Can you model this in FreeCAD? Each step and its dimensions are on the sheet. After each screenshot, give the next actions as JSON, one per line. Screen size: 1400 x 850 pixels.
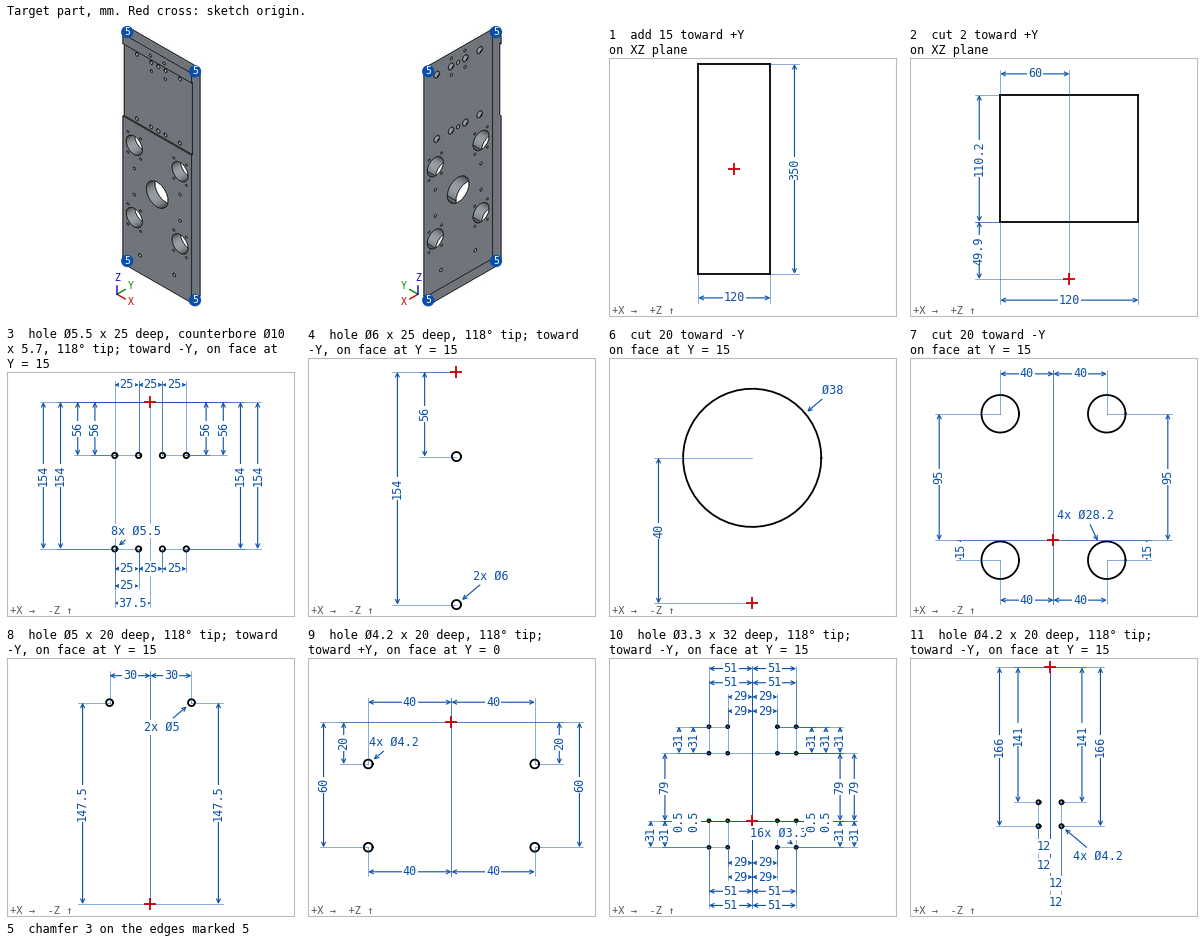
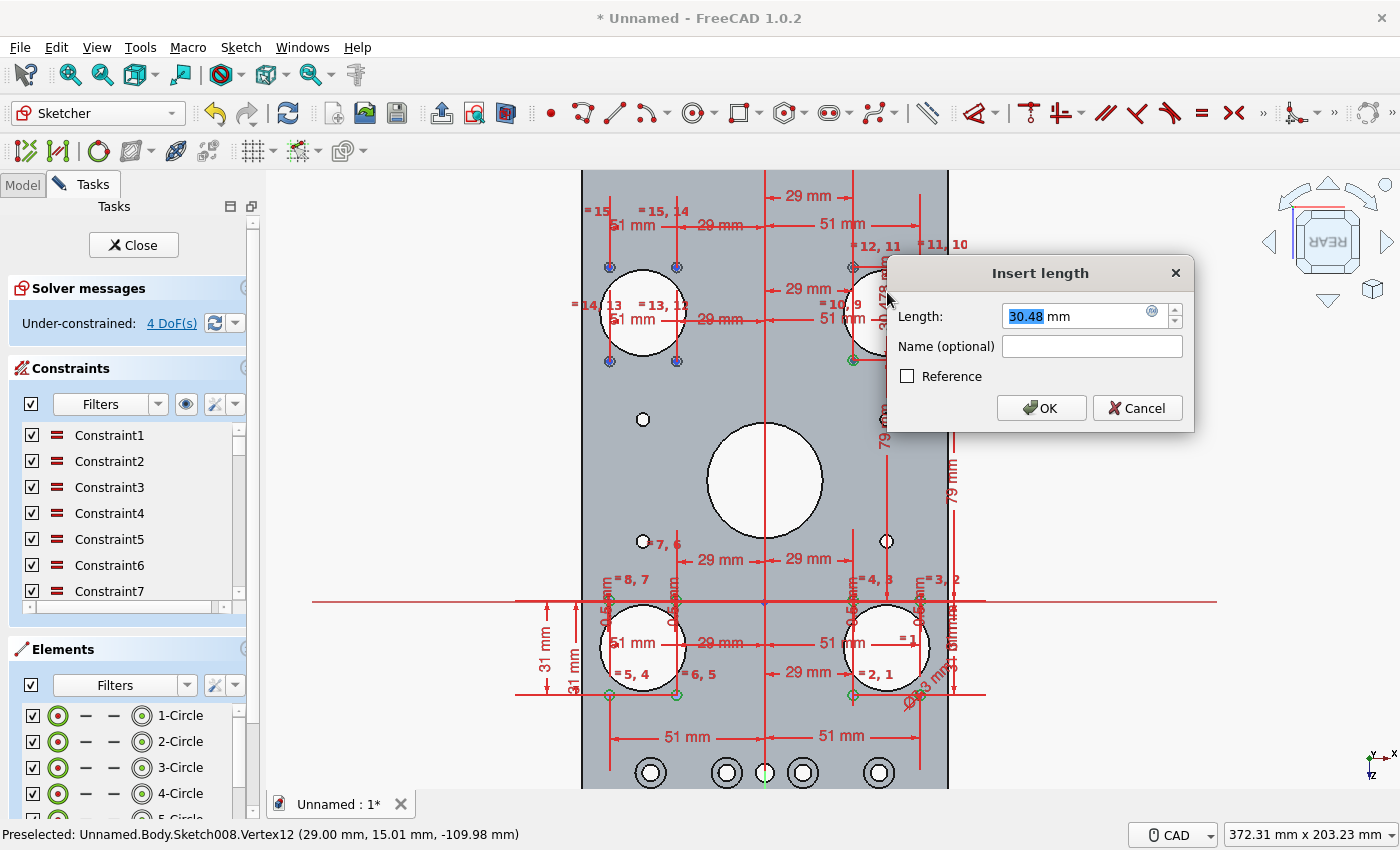
{"action": "type", "text": "31"}
{"action": "key", "text": "Return"}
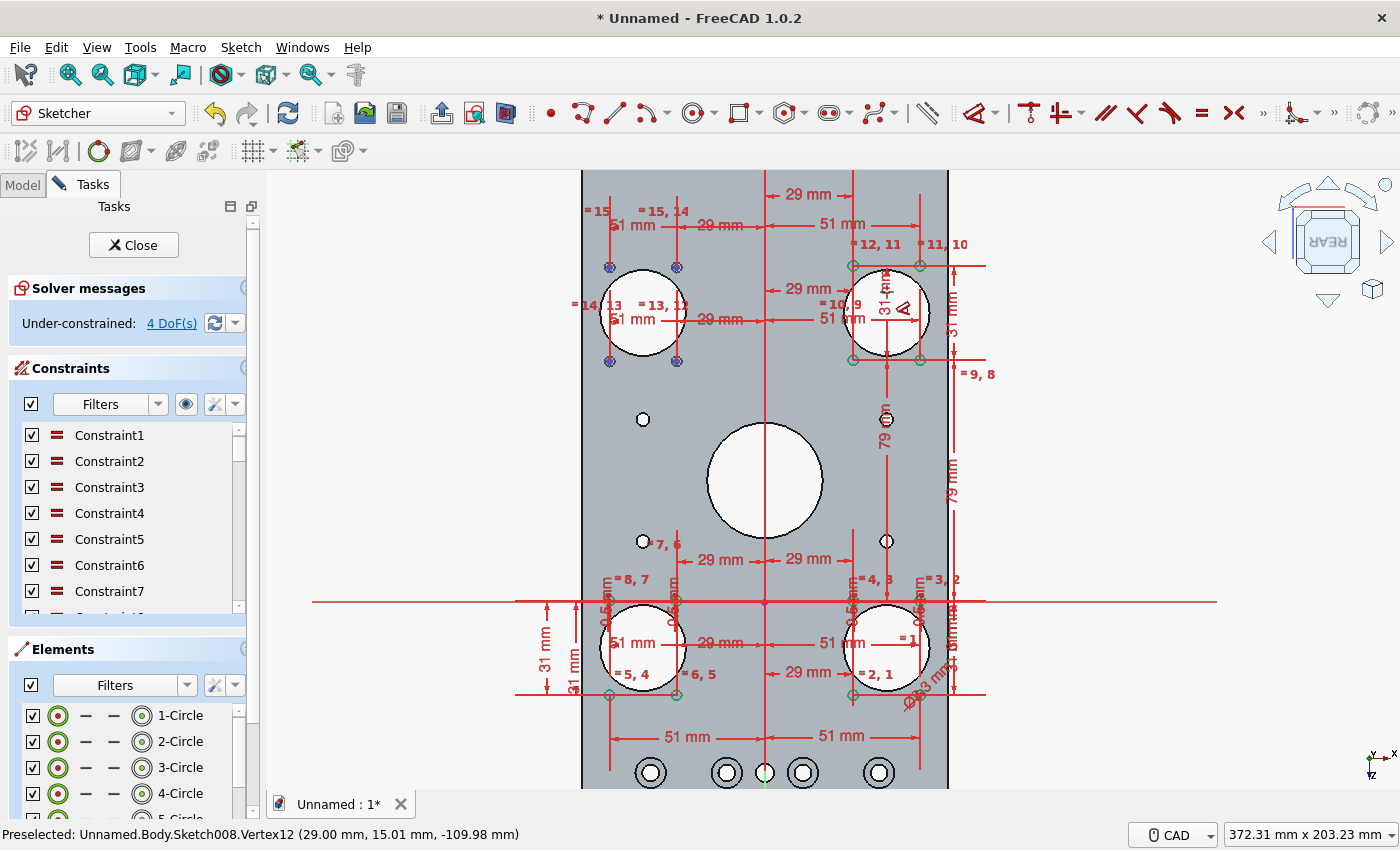
{"action": "left_click", "coordinate": [853, 266]}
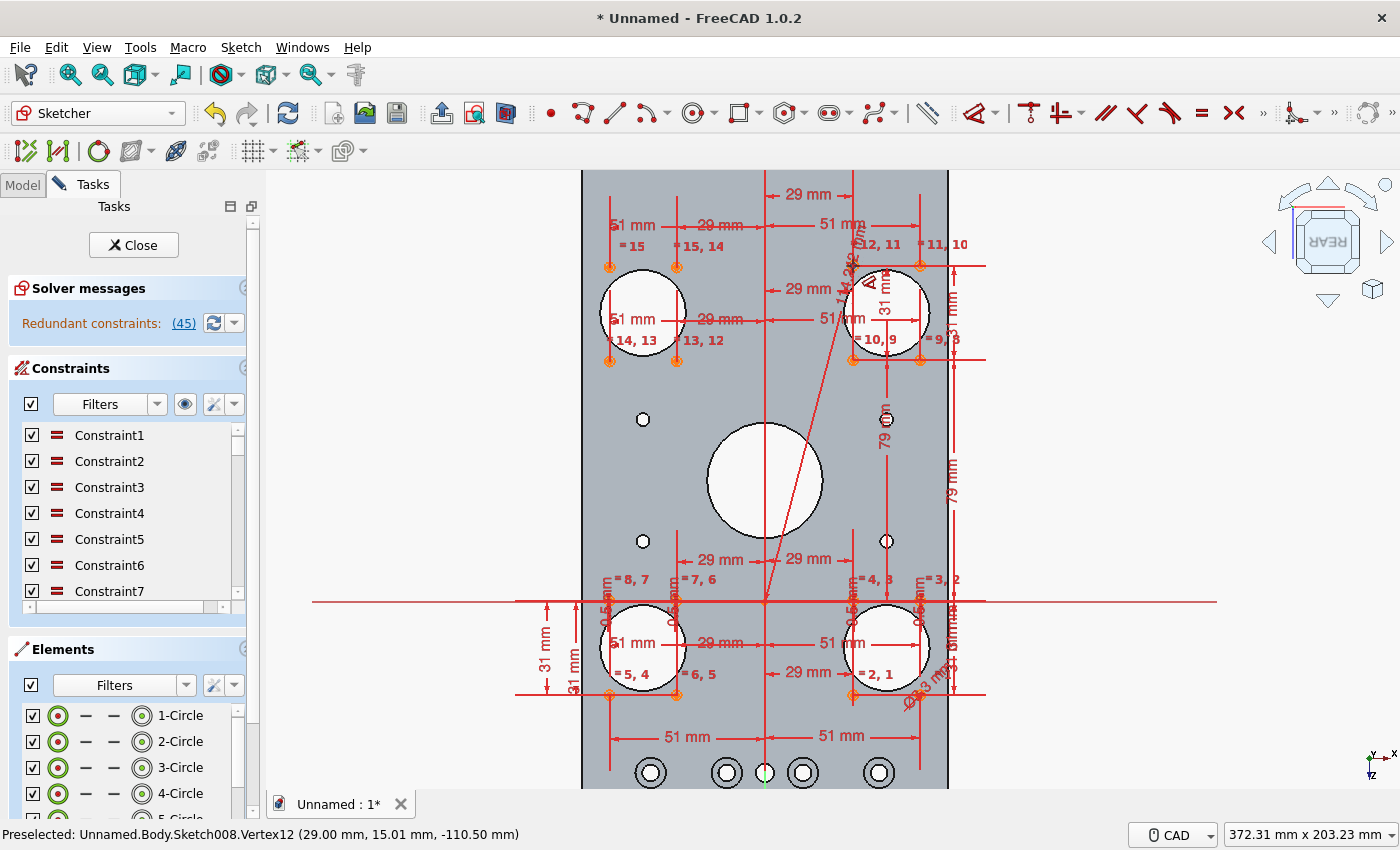
{"action": "left_click", "coordinate": [677, 361]}
{"action": "left_click", "coordinate": [887, 347]}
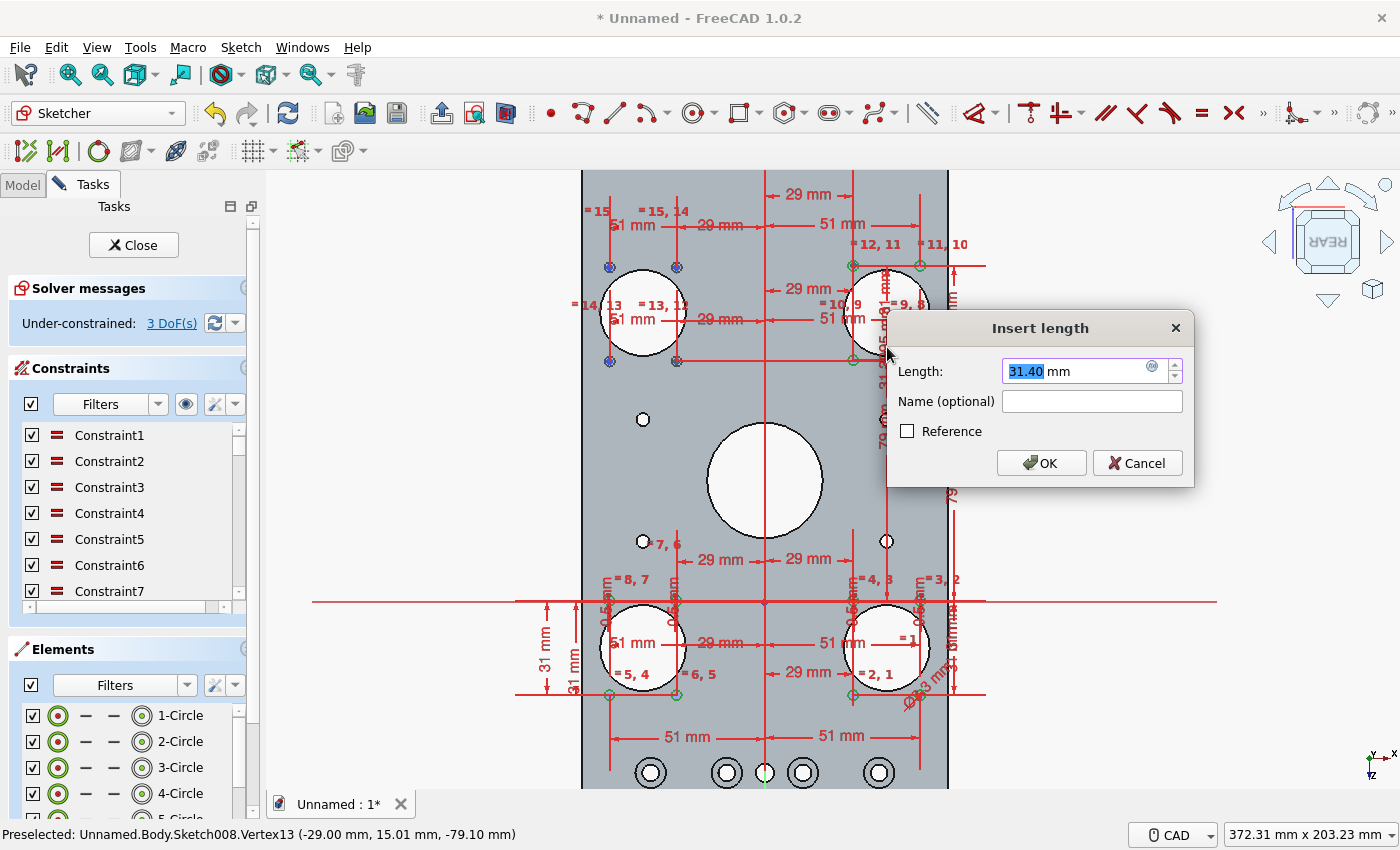
{"action": "type", "text": "31"}
{"action": "key", "text": "Return"}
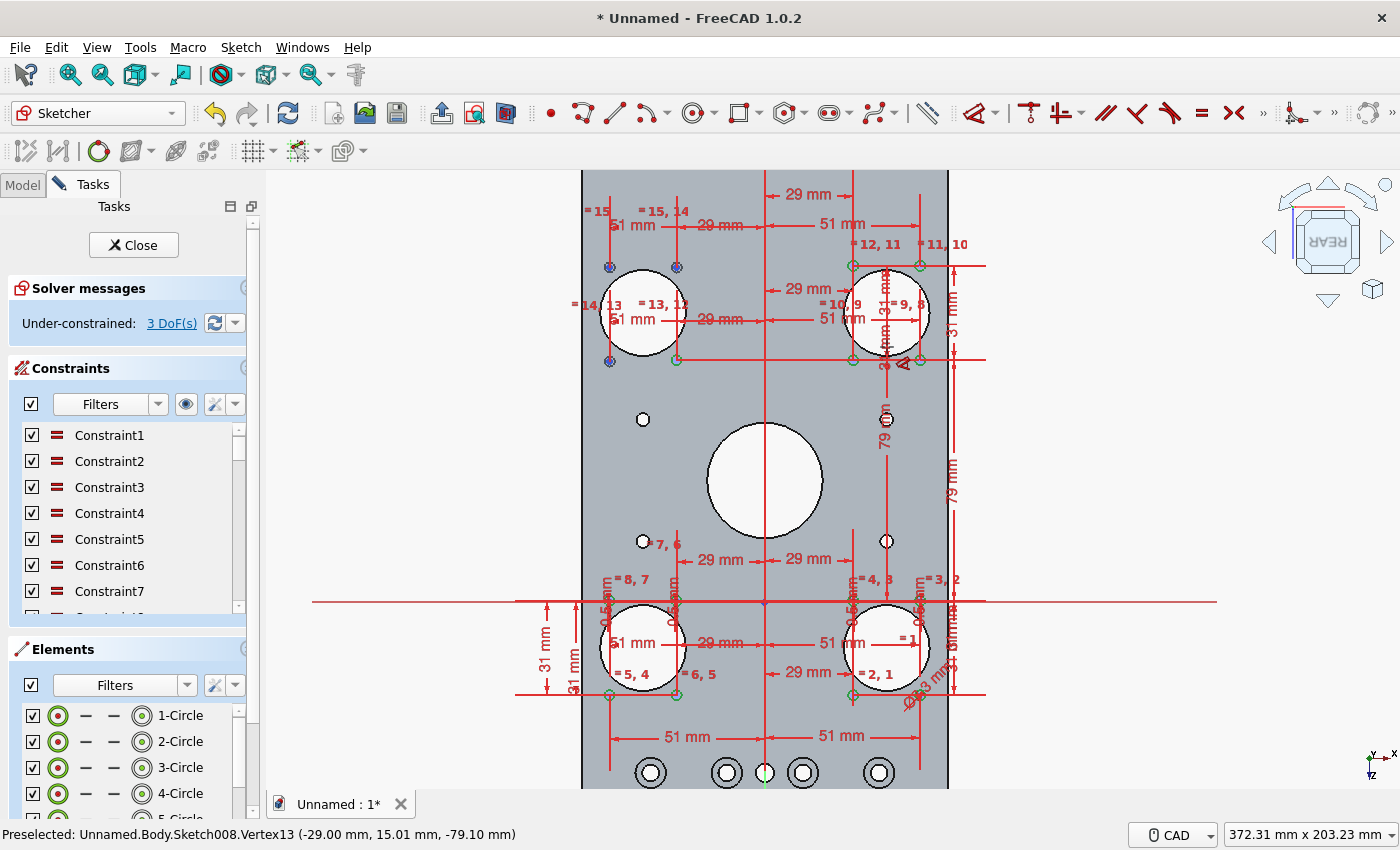
{"action": "left_click", "coordinate": [610, 601]}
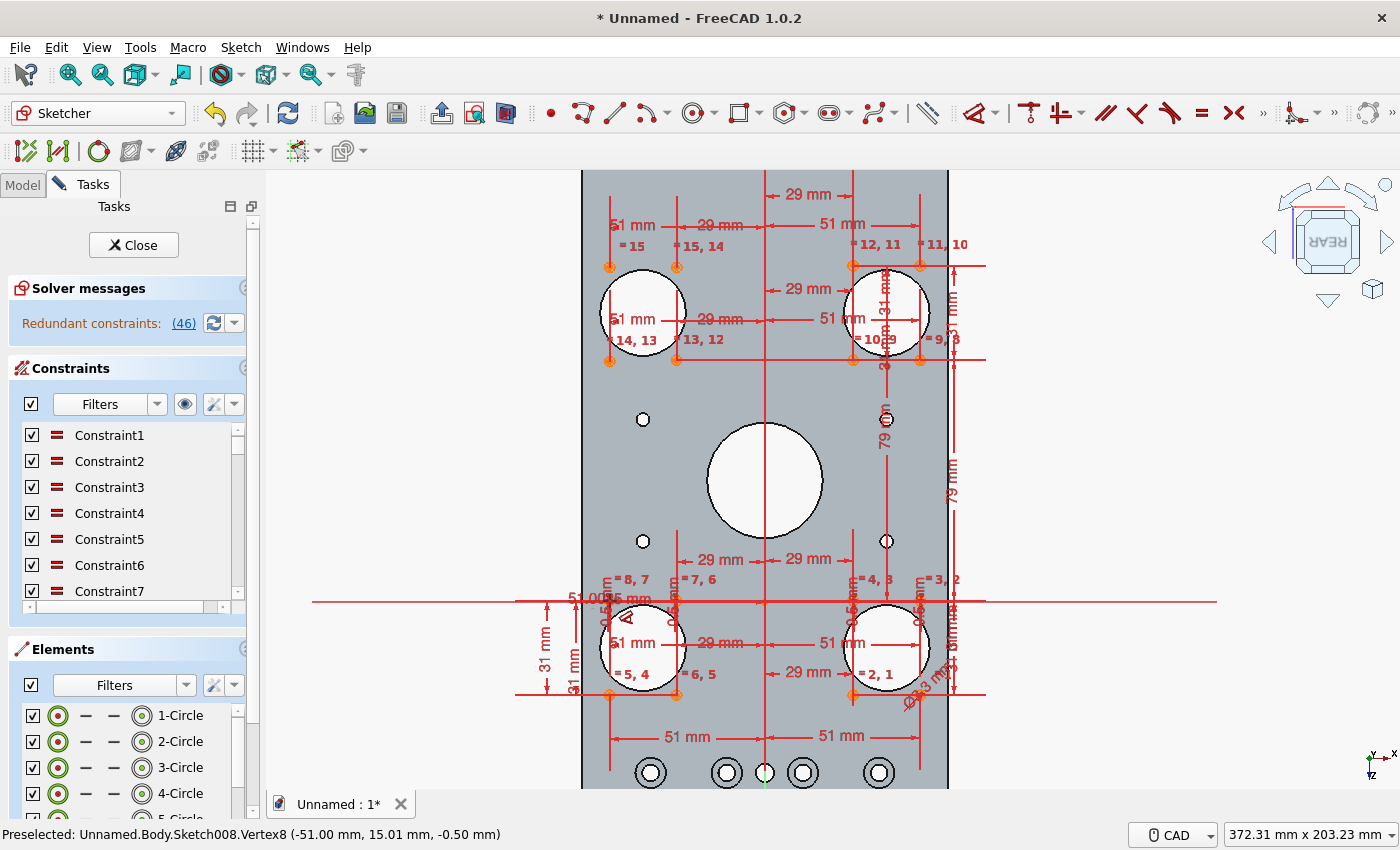
{"action": "left_click", "coordinate": [610, 362]}
{"action": "left_click", "coordinate": [576, 481]}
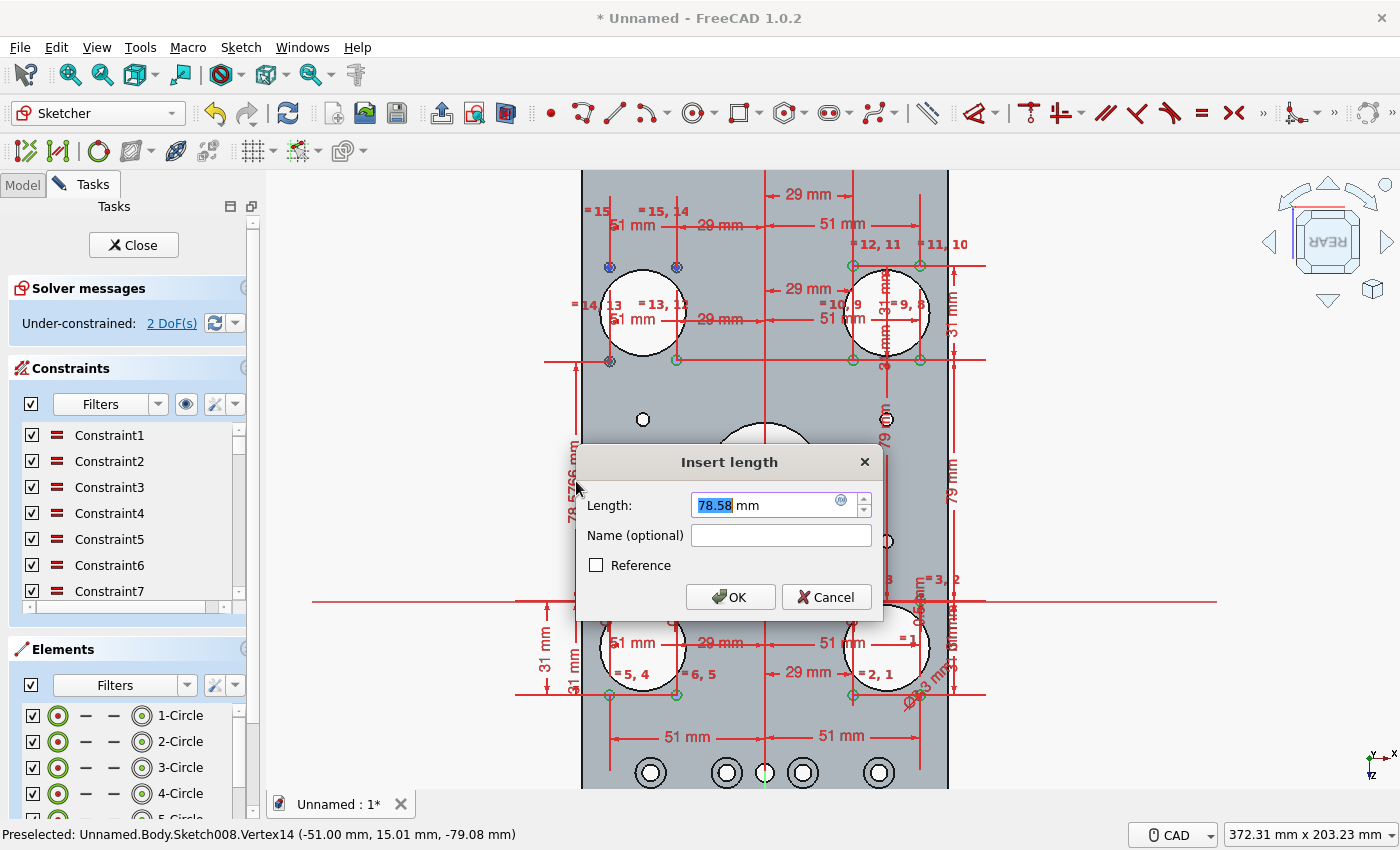
{"action": "type", "text": "79"}
{"action": "key", "text": "Return"}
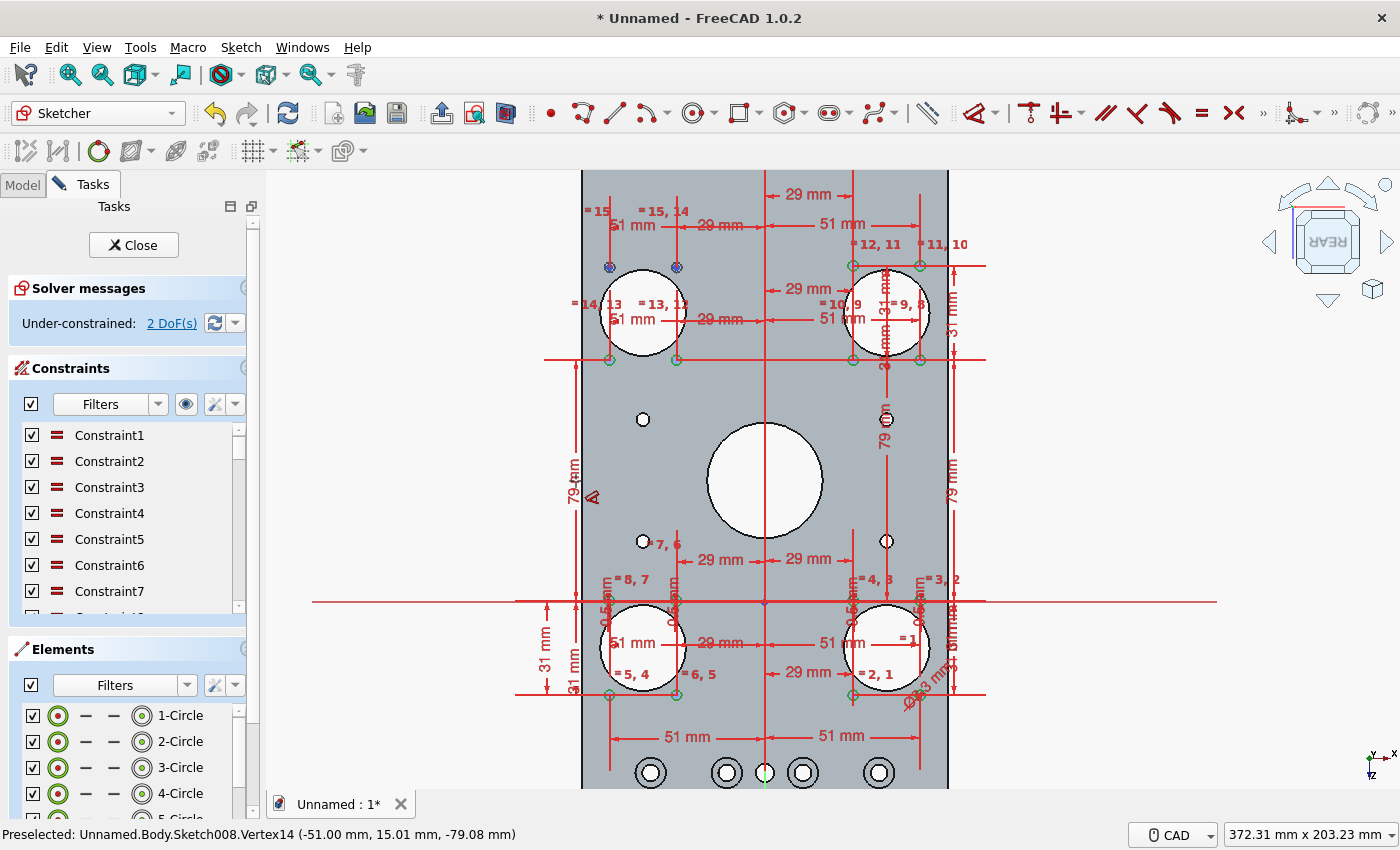
{"action": "left_click", "coordinate": [677, 360]}